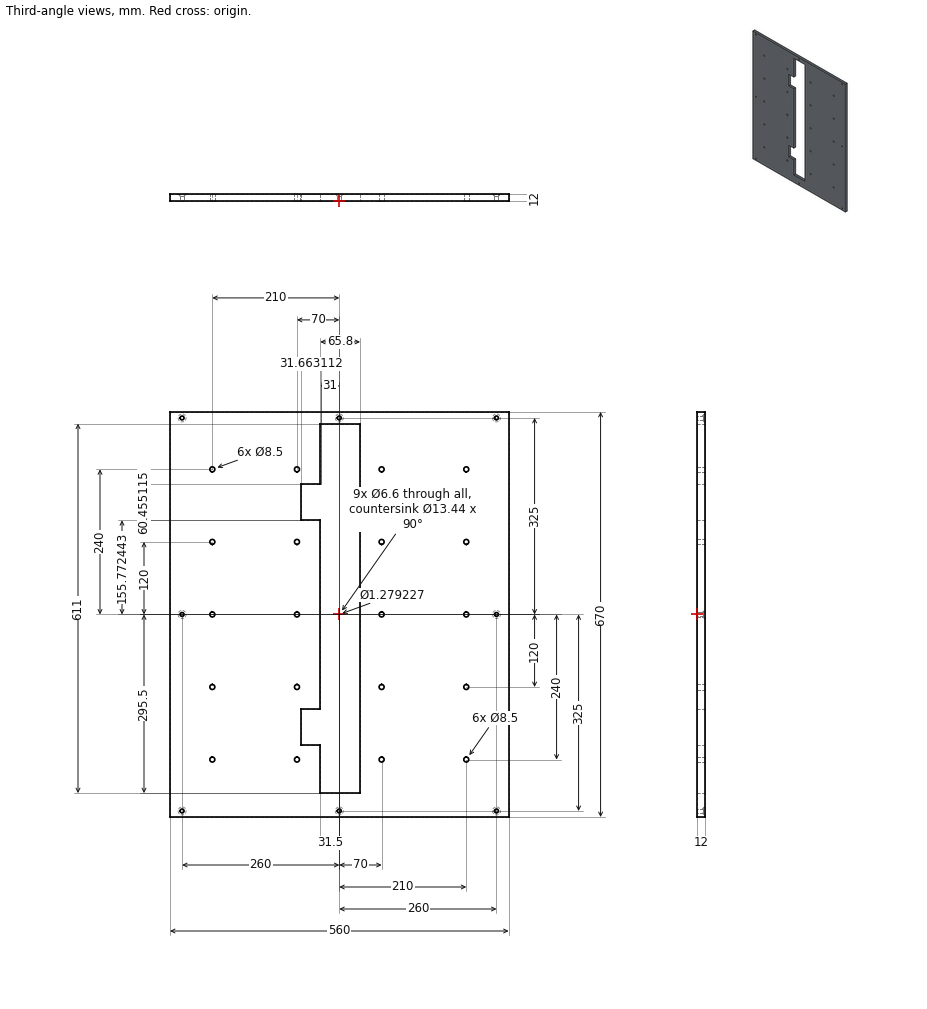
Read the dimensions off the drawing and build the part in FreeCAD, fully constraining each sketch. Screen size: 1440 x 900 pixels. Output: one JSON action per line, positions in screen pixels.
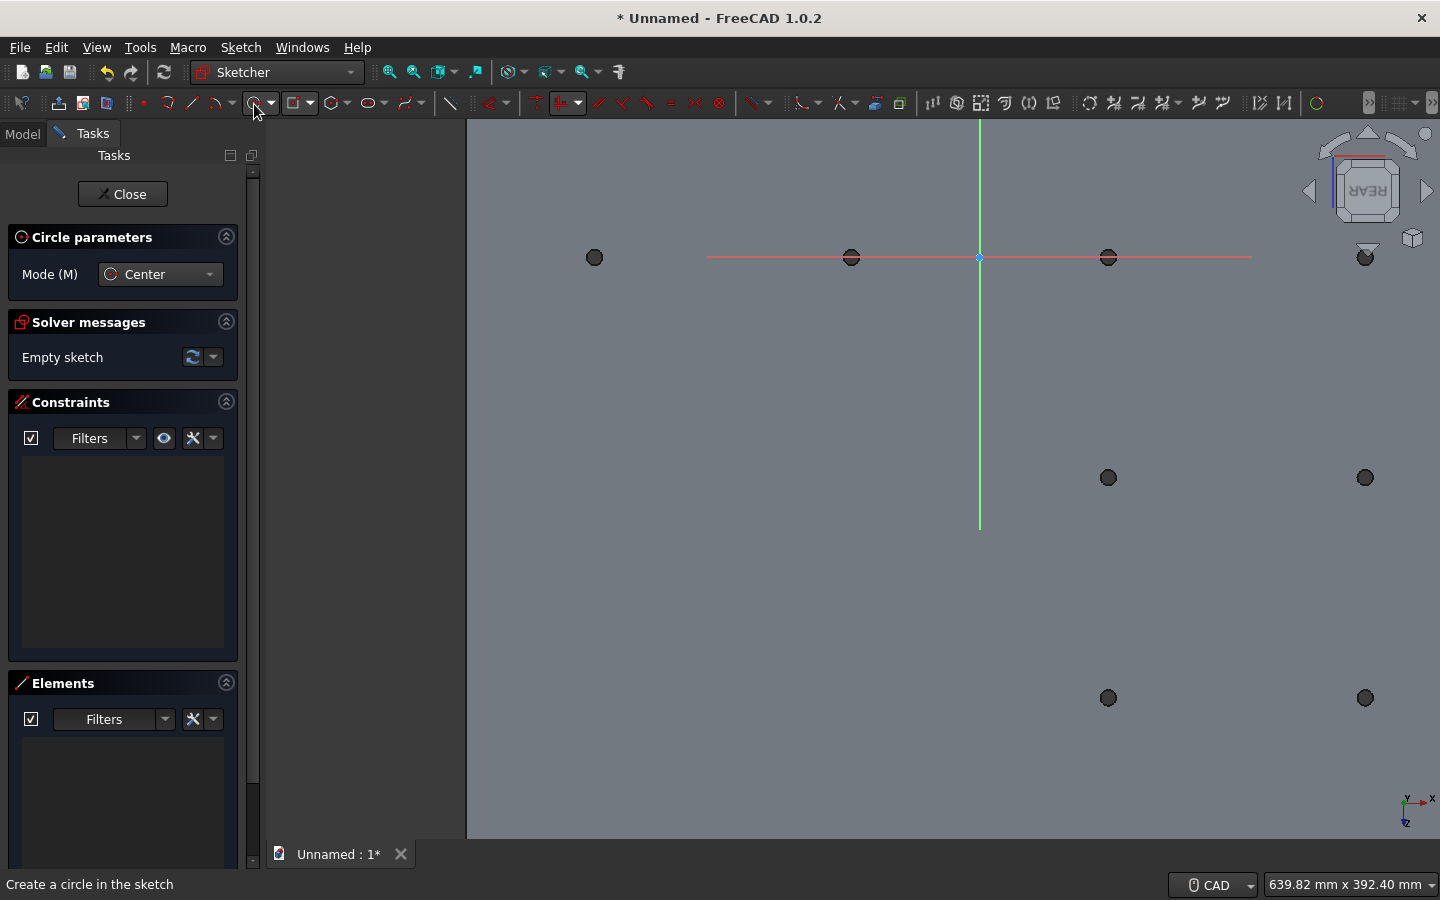
{"action": "scroll", "coordinate": [595, 698], "scroll_direction": "up", "scroll_amount": 6}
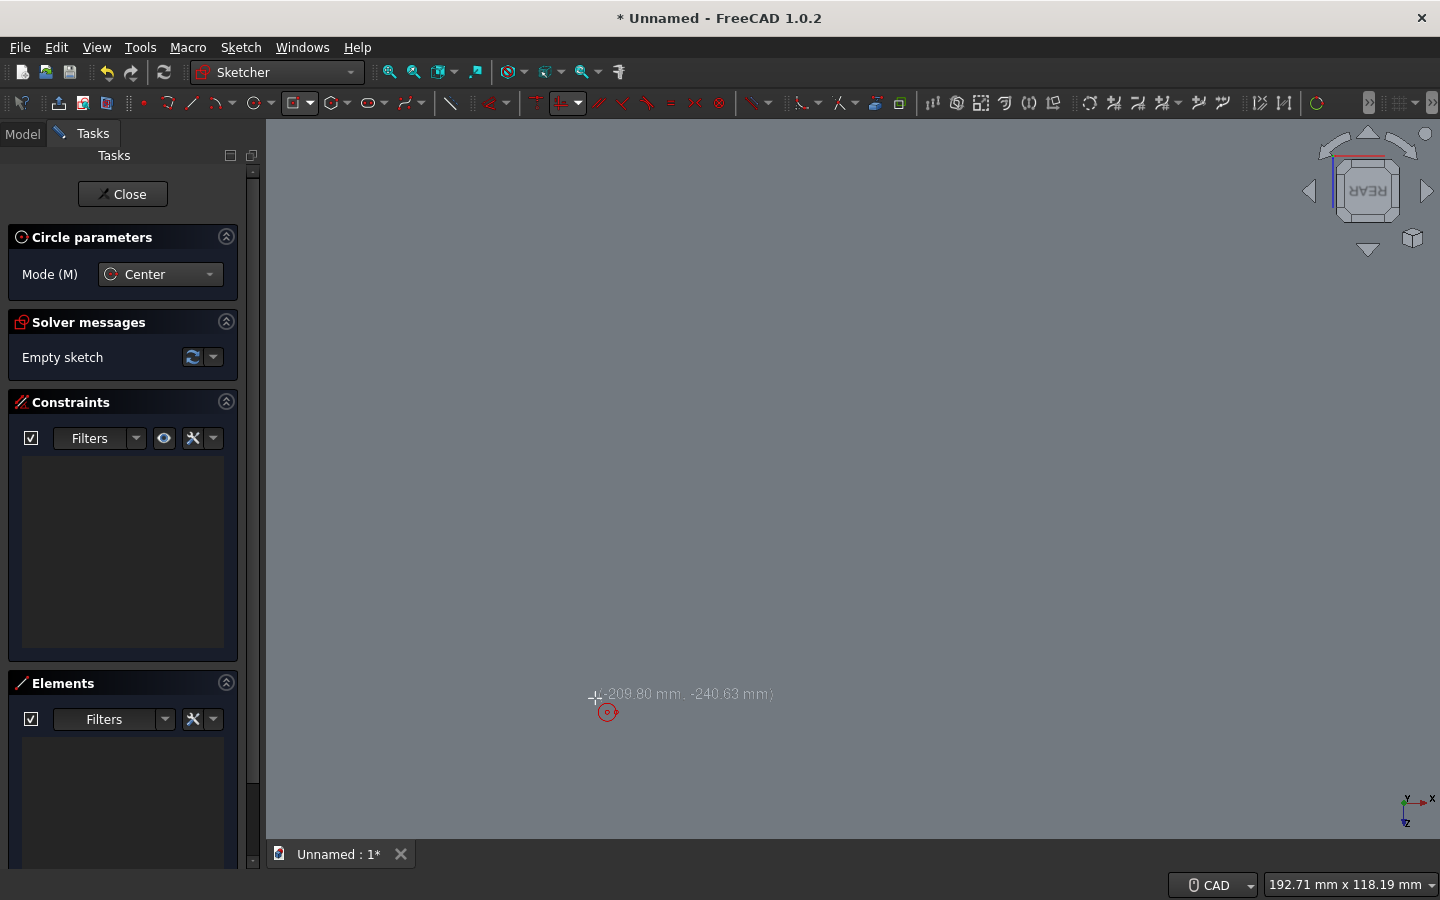
{"action": "left_click", "coordinate": [593, 696]}
{"action": "left_click", "coordinate": [611, 677]}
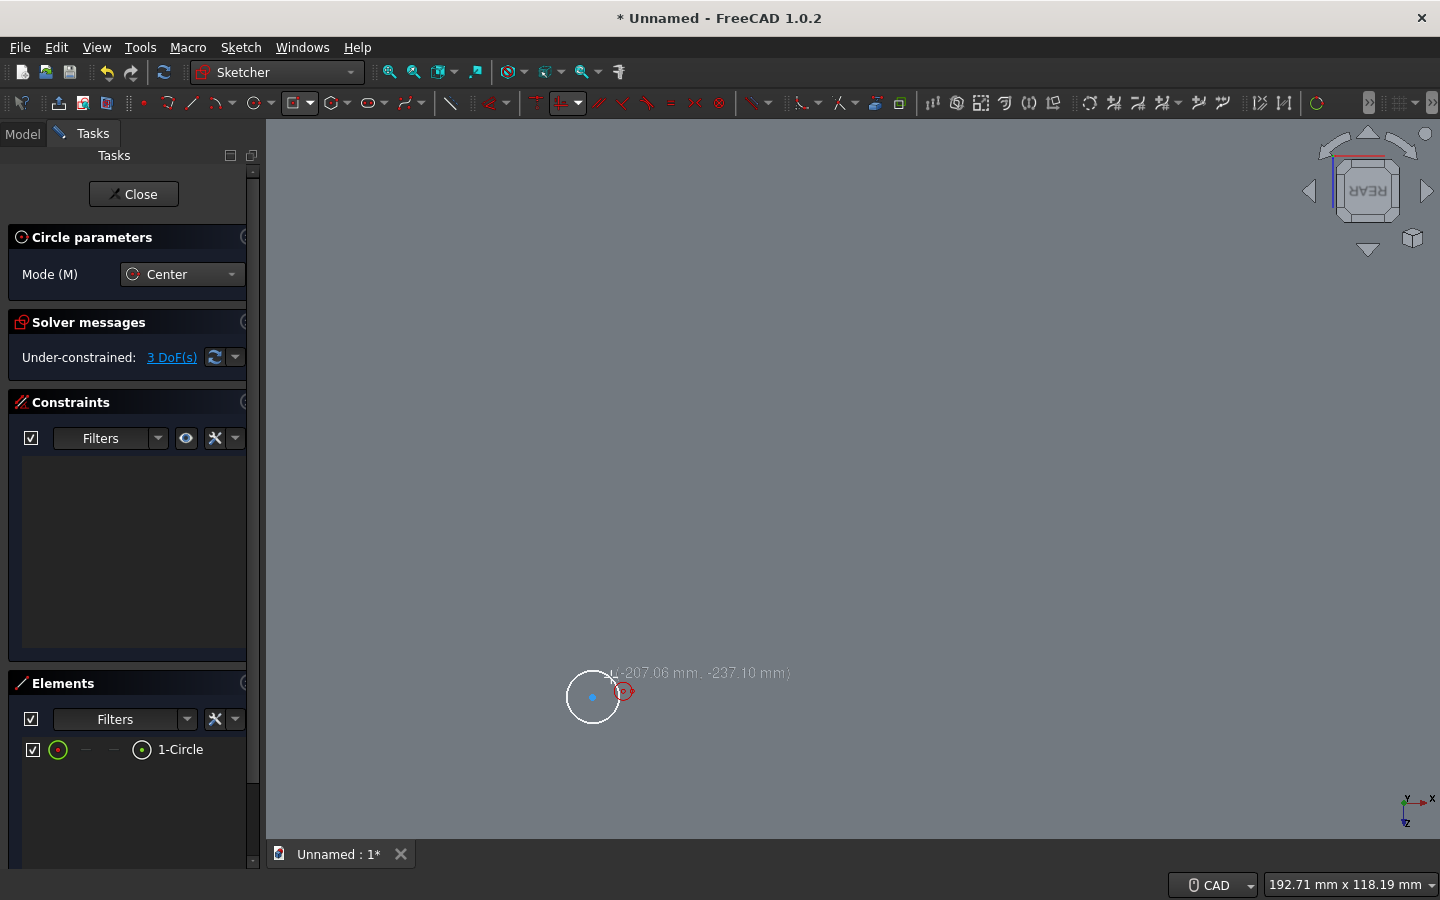
{"action": "scroll", "coordinate": [596, 701], "scroll_direction": "down", "scroll_amount": 6}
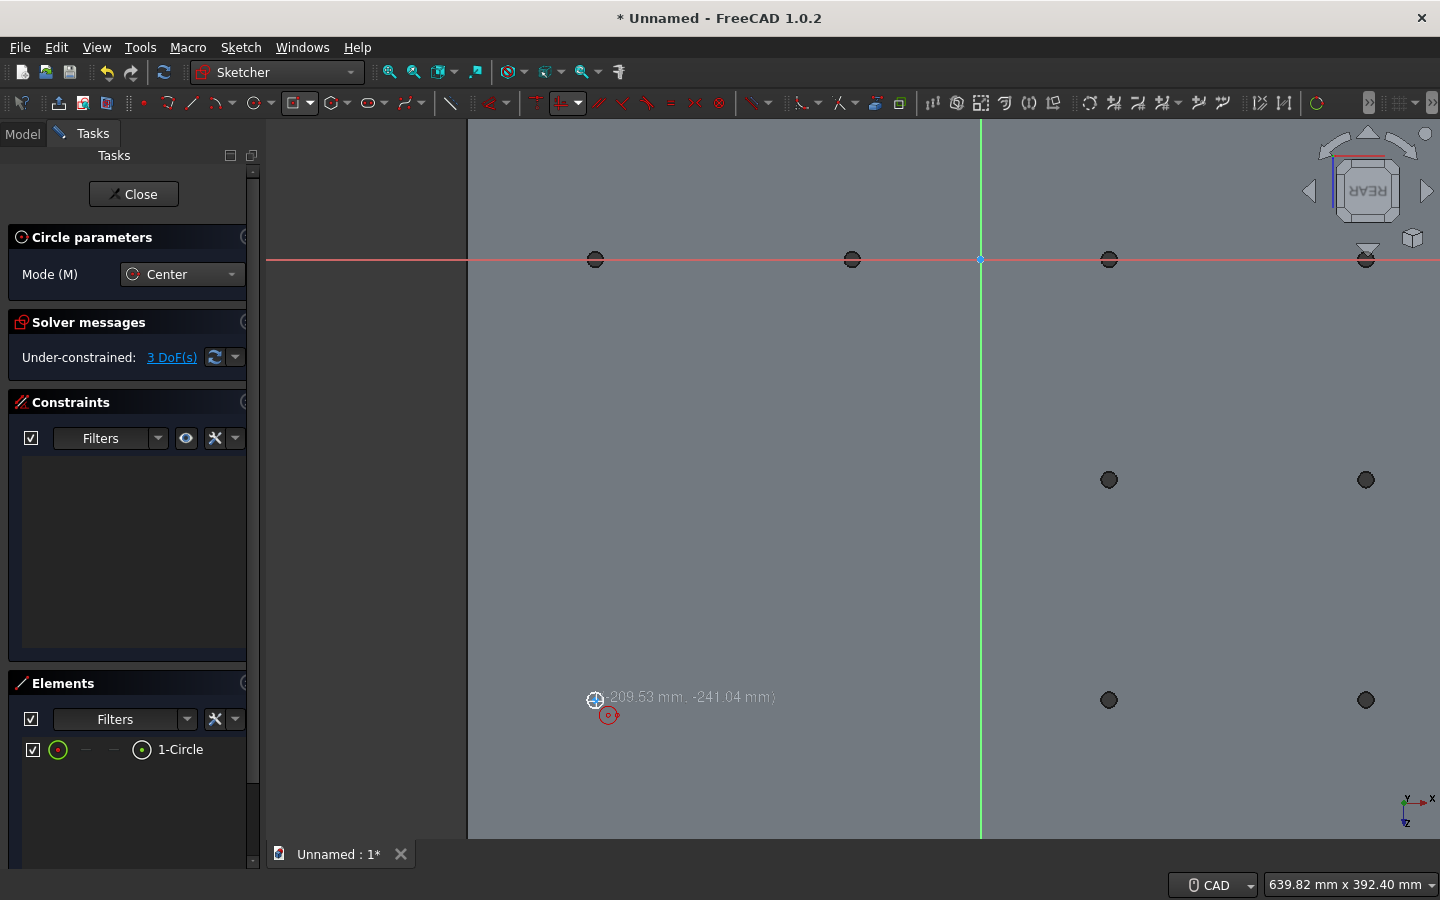
{"action": "scroll", "coordinate": [852, 700], "scroll_direction": "up", "scroll_amount": 6}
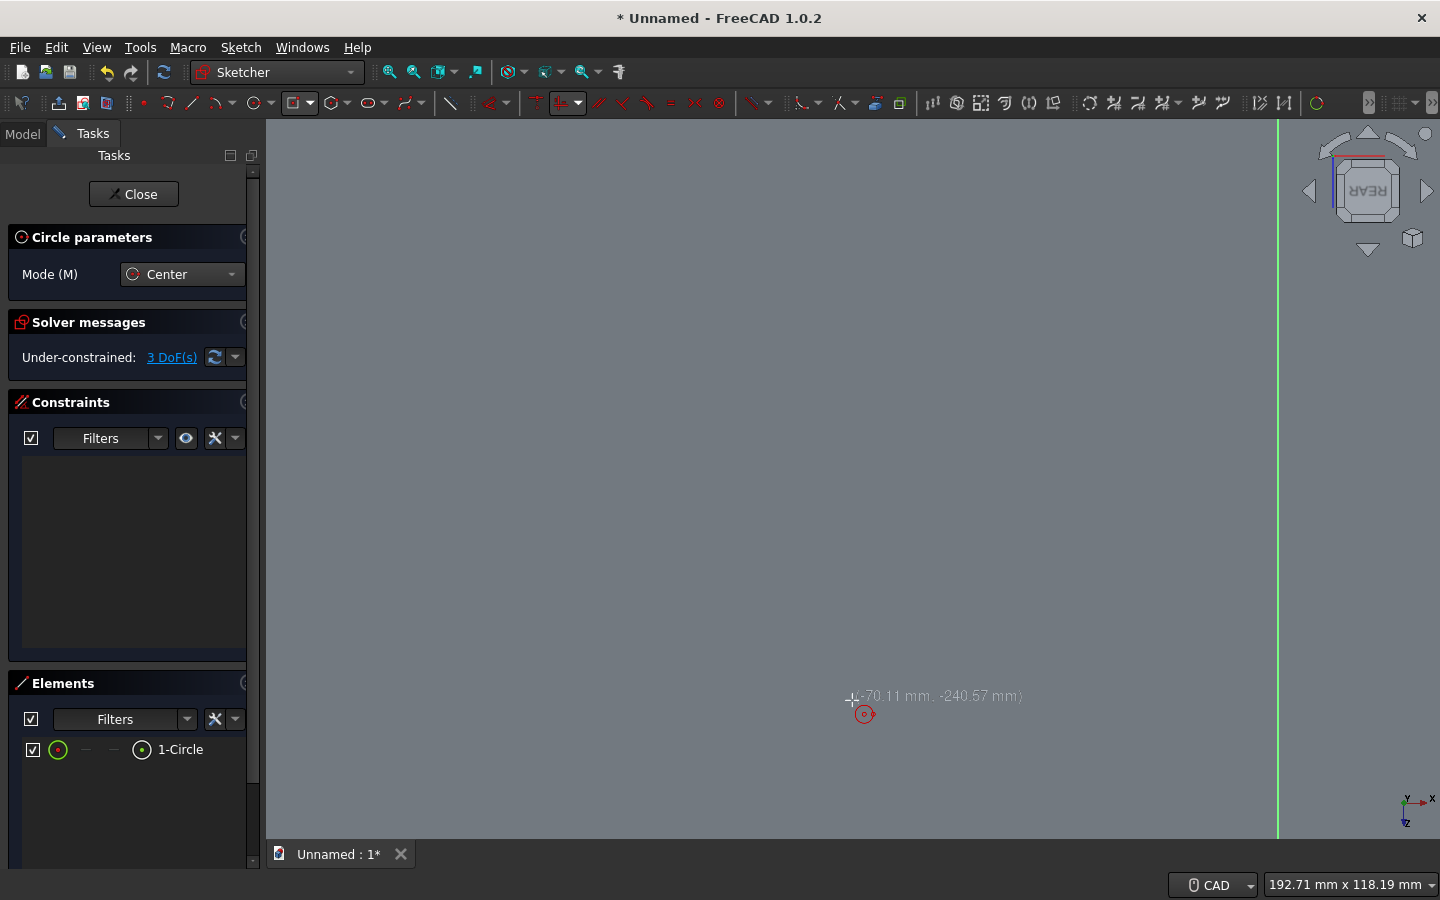
{"action": "left_click", "coordinate": [852, 698]}
{"action": "left_click", "coordinate": [870, 680]}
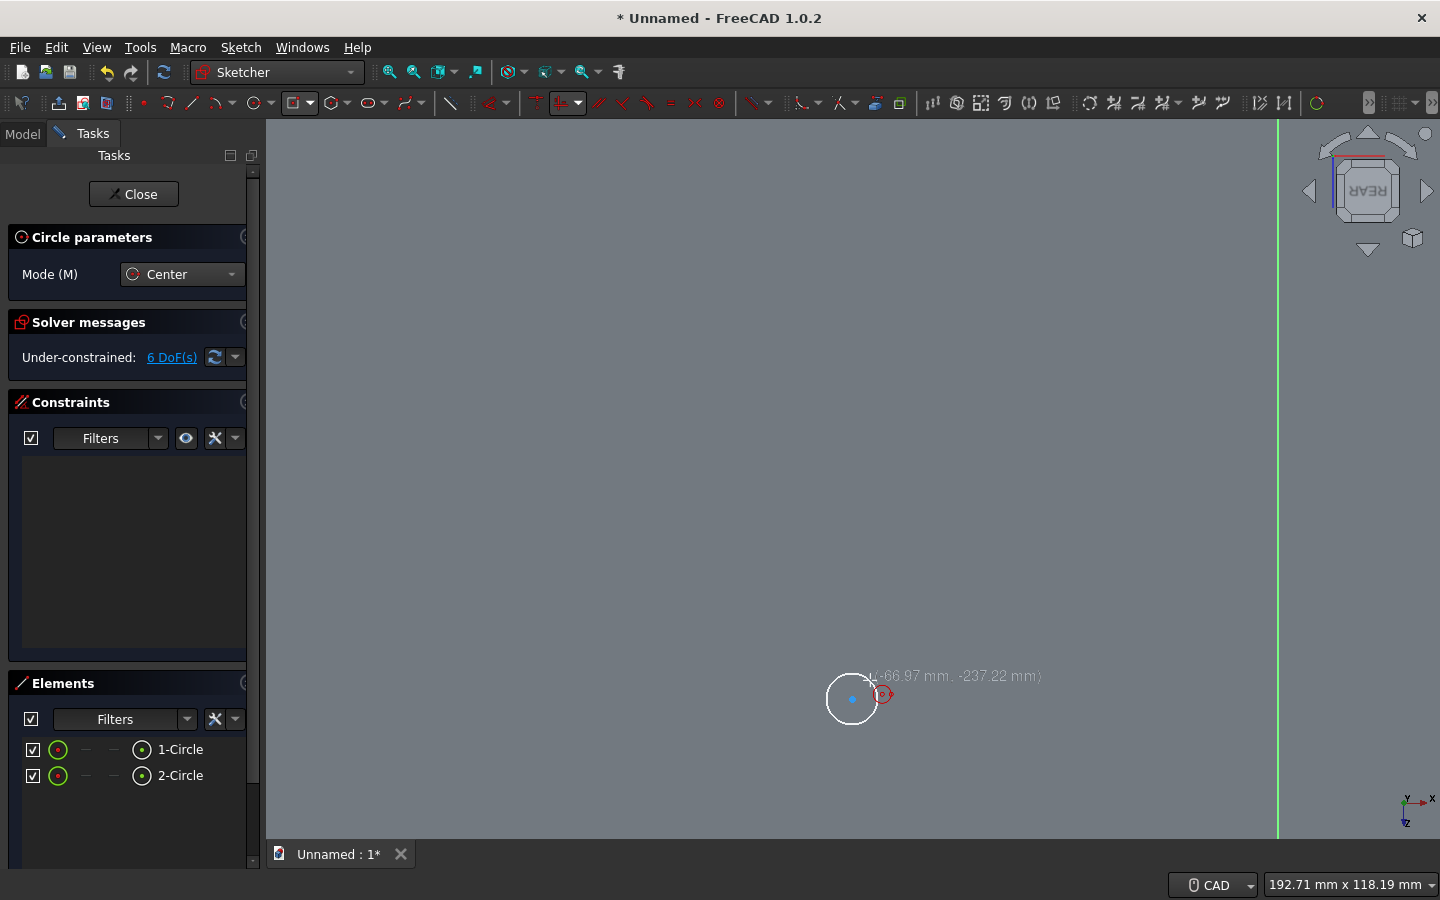
{"action": "scroll", "coordinate": [852, 700], "scroll_direction": "down", "scroll_amount": 6}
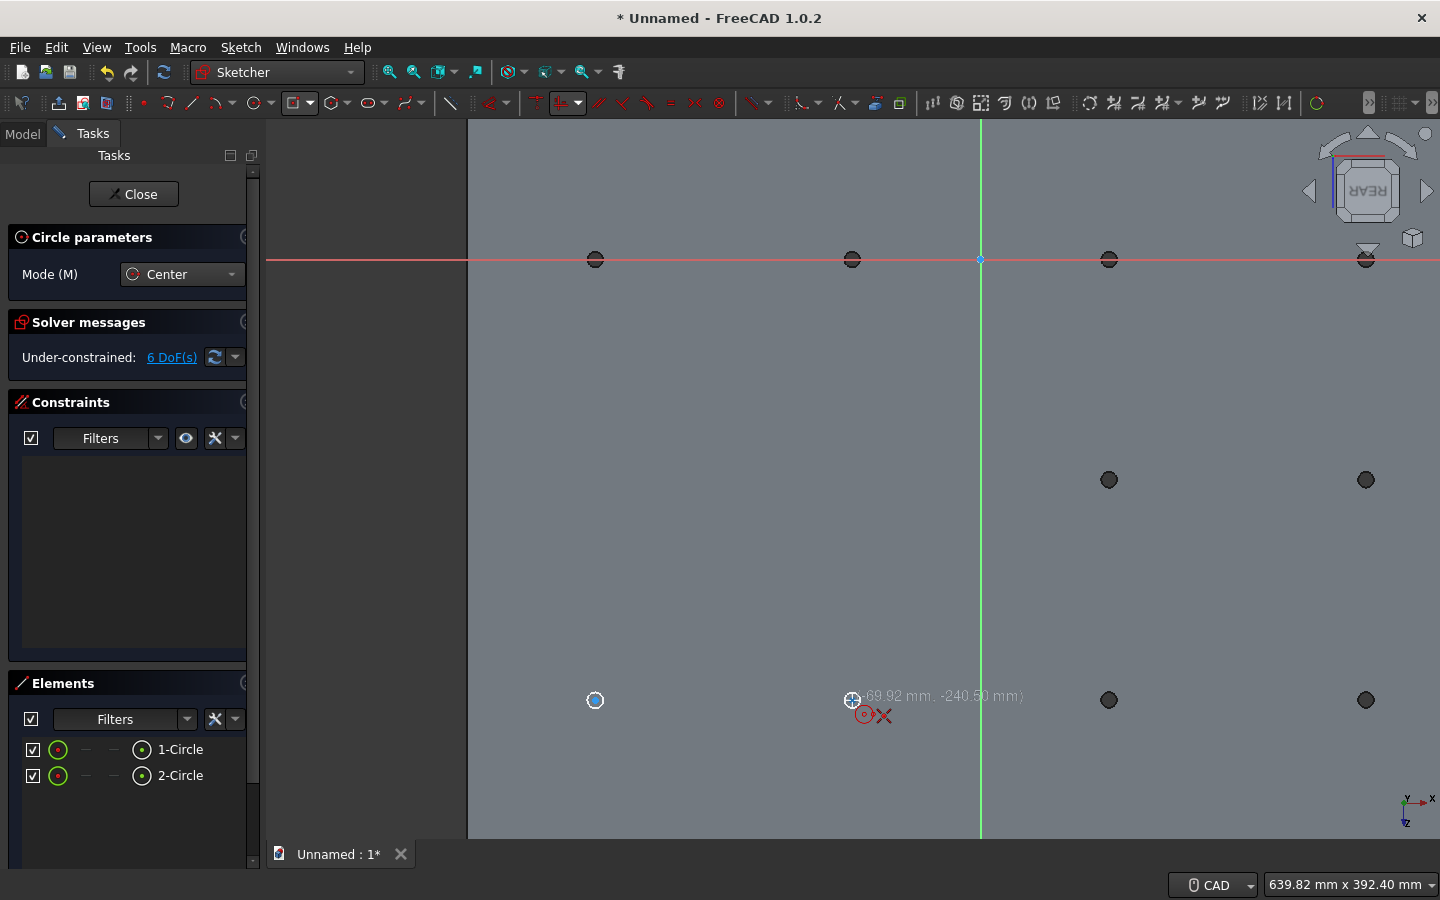
{"action": "scroll", "coordinate": [595, 480], "scroll_direction": "up", "scroll_amount": 6}